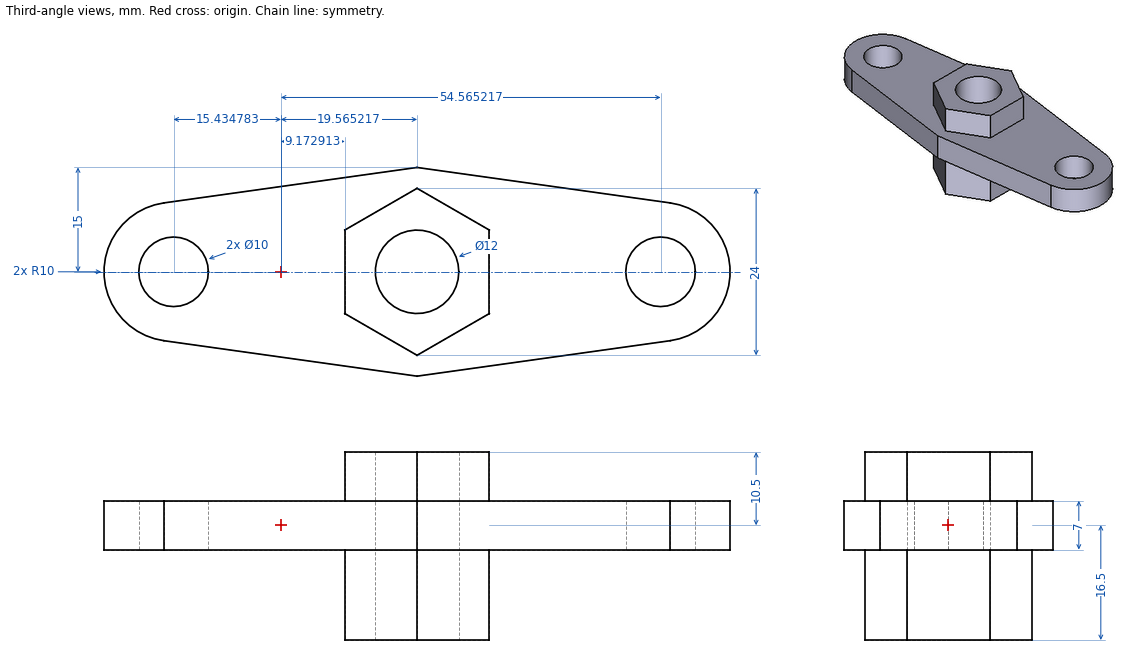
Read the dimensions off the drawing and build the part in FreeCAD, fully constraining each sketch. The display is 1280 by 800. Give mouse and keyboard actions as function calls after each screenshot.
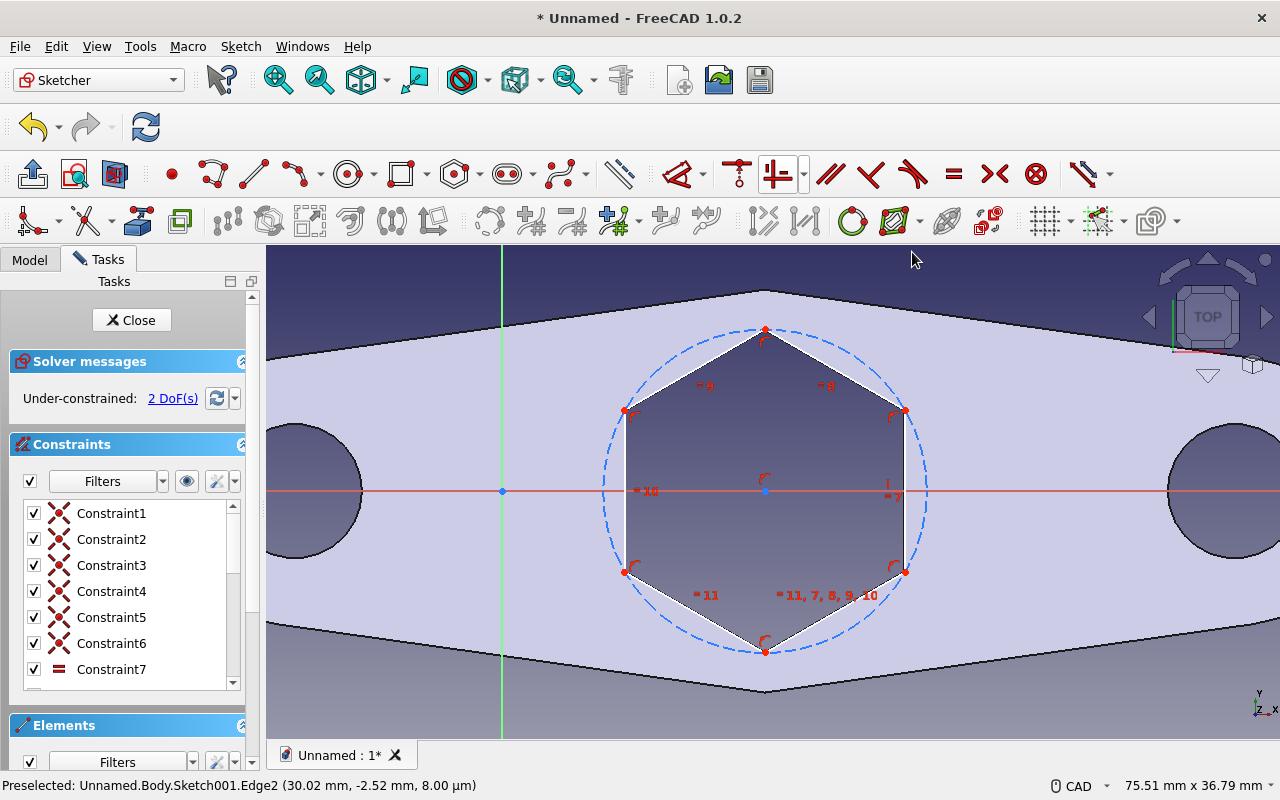
click(676, 174)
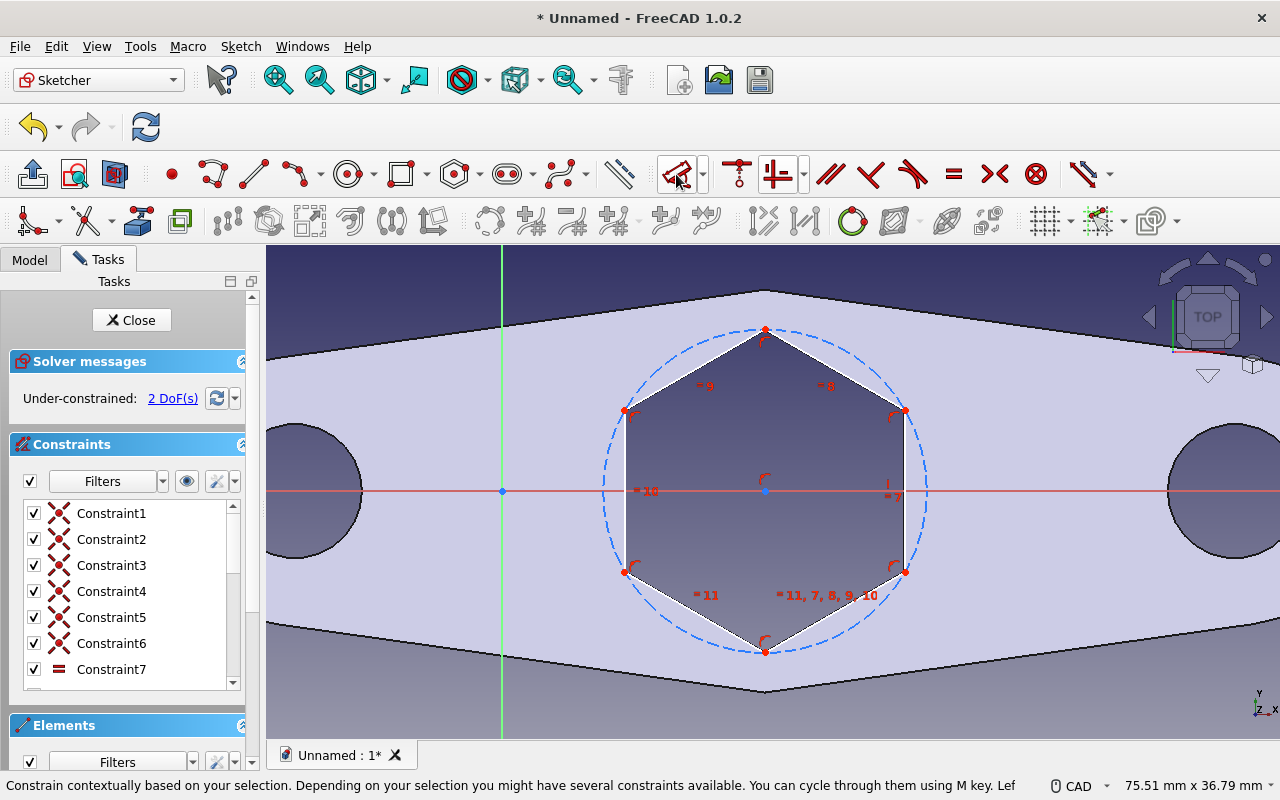
click(765, 653)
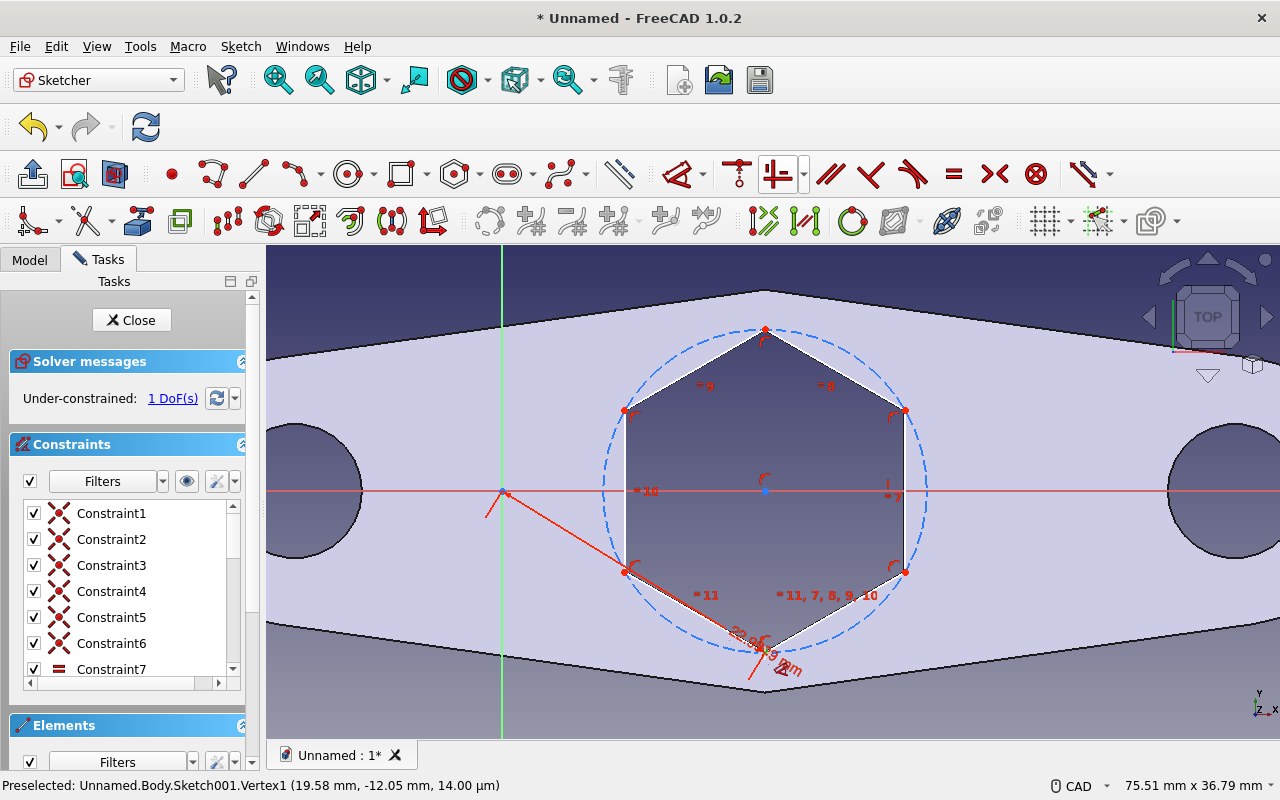
click(765, 329)
click(799, 417)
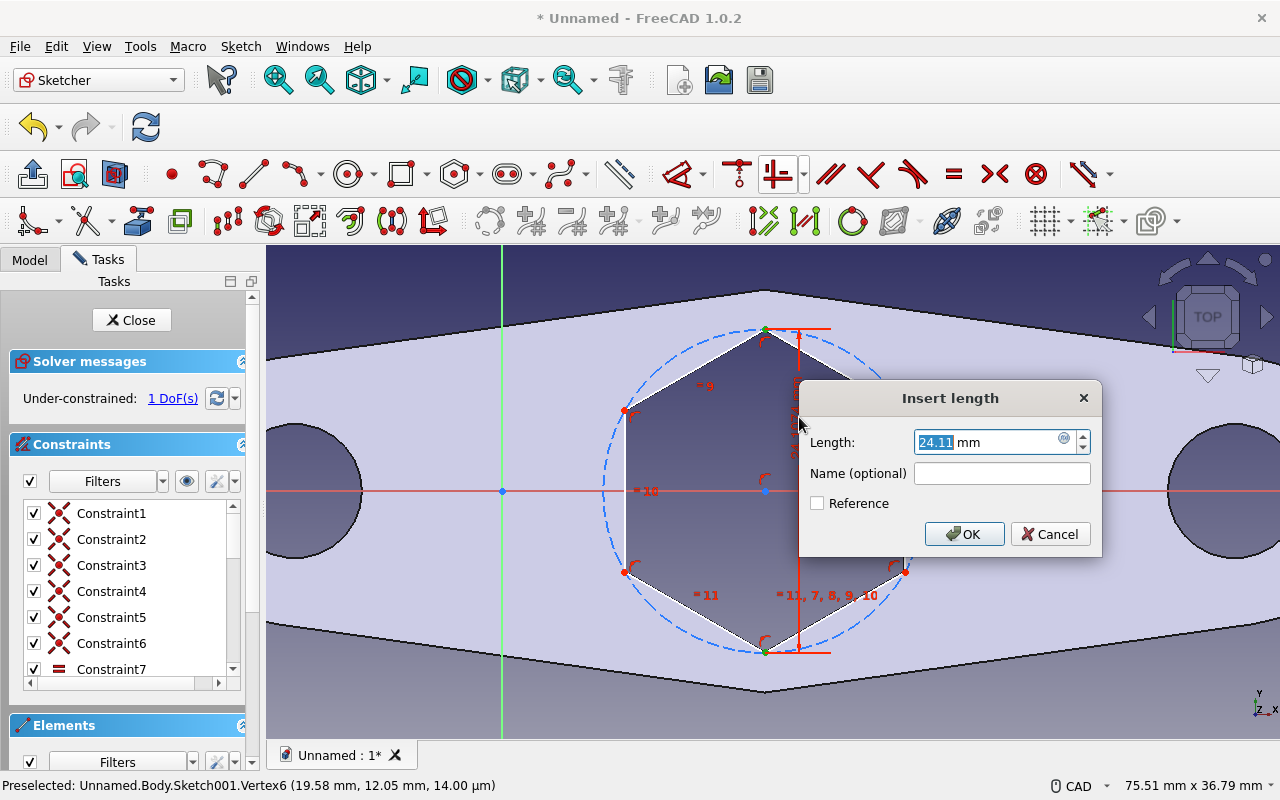
text(24)
key(Return)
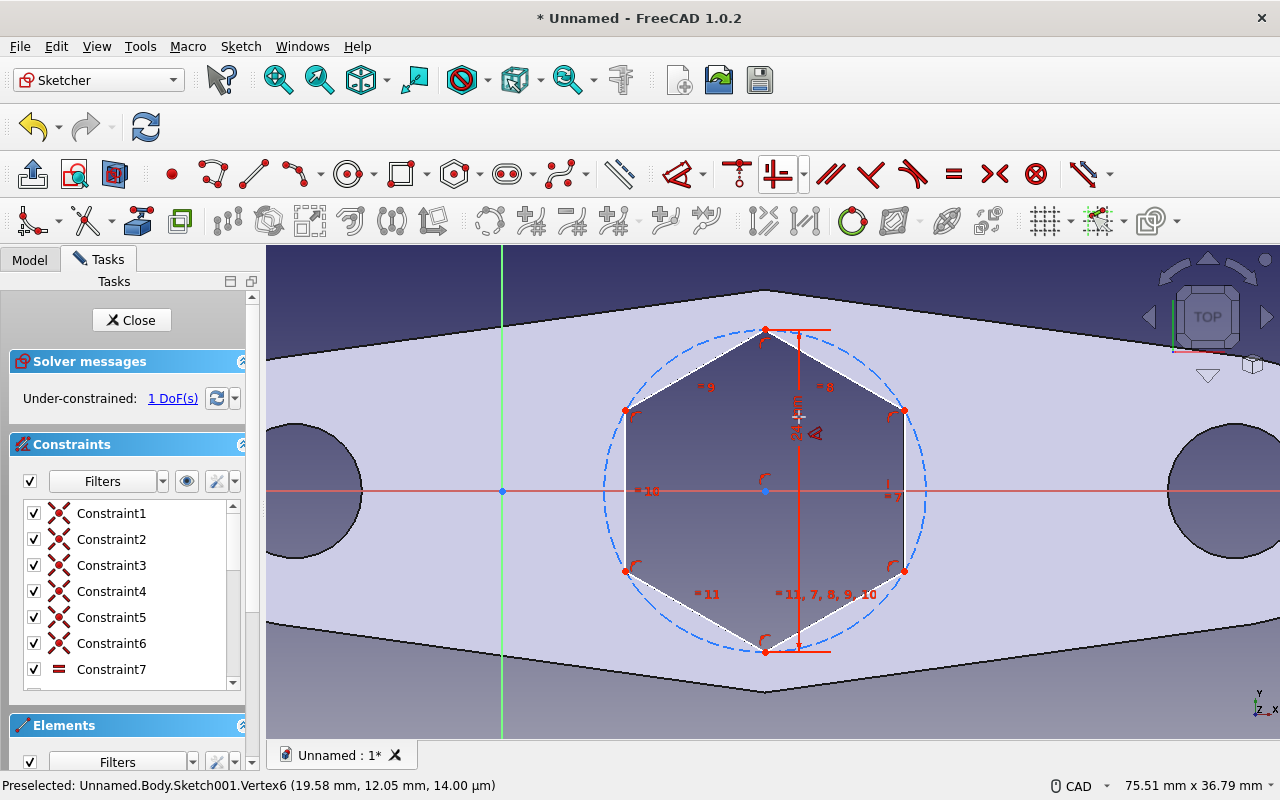
click(625, 411)
click(564, 377)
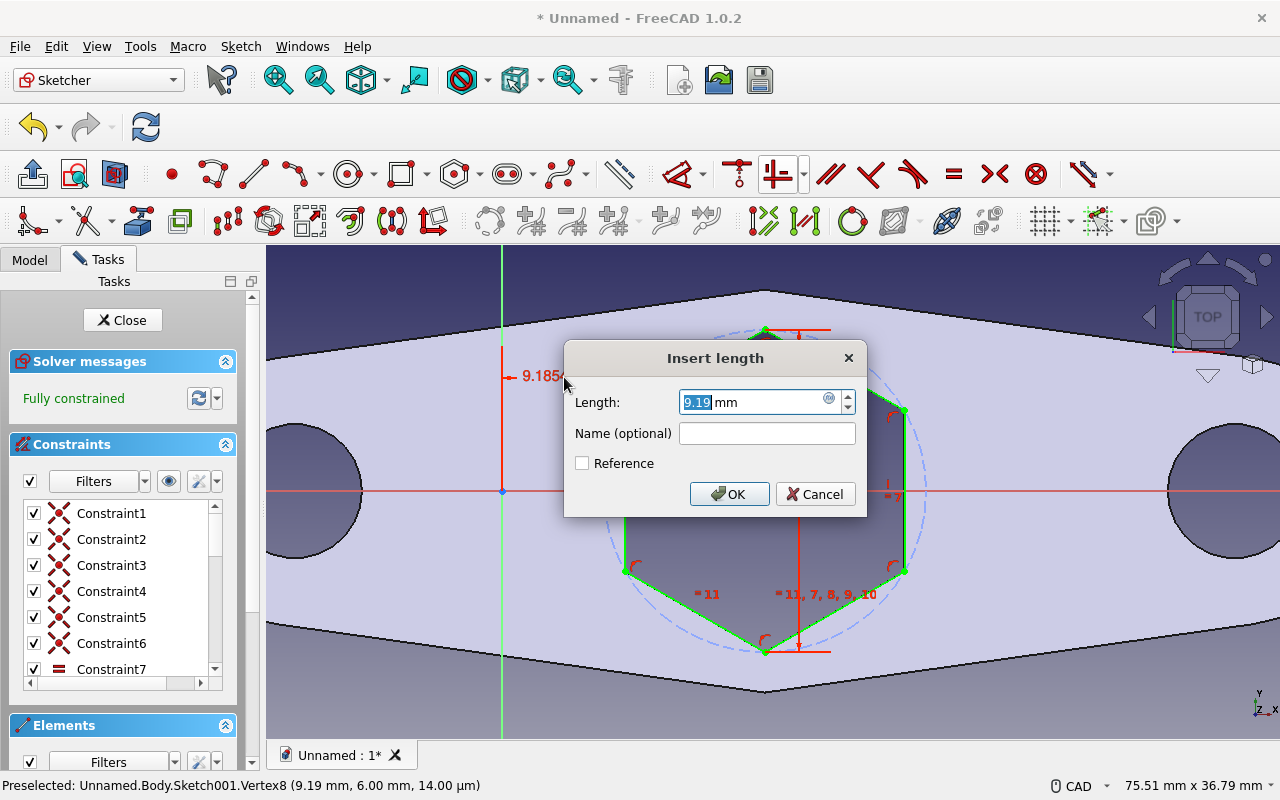
text(9.172913)
key(Return)
key(Escape)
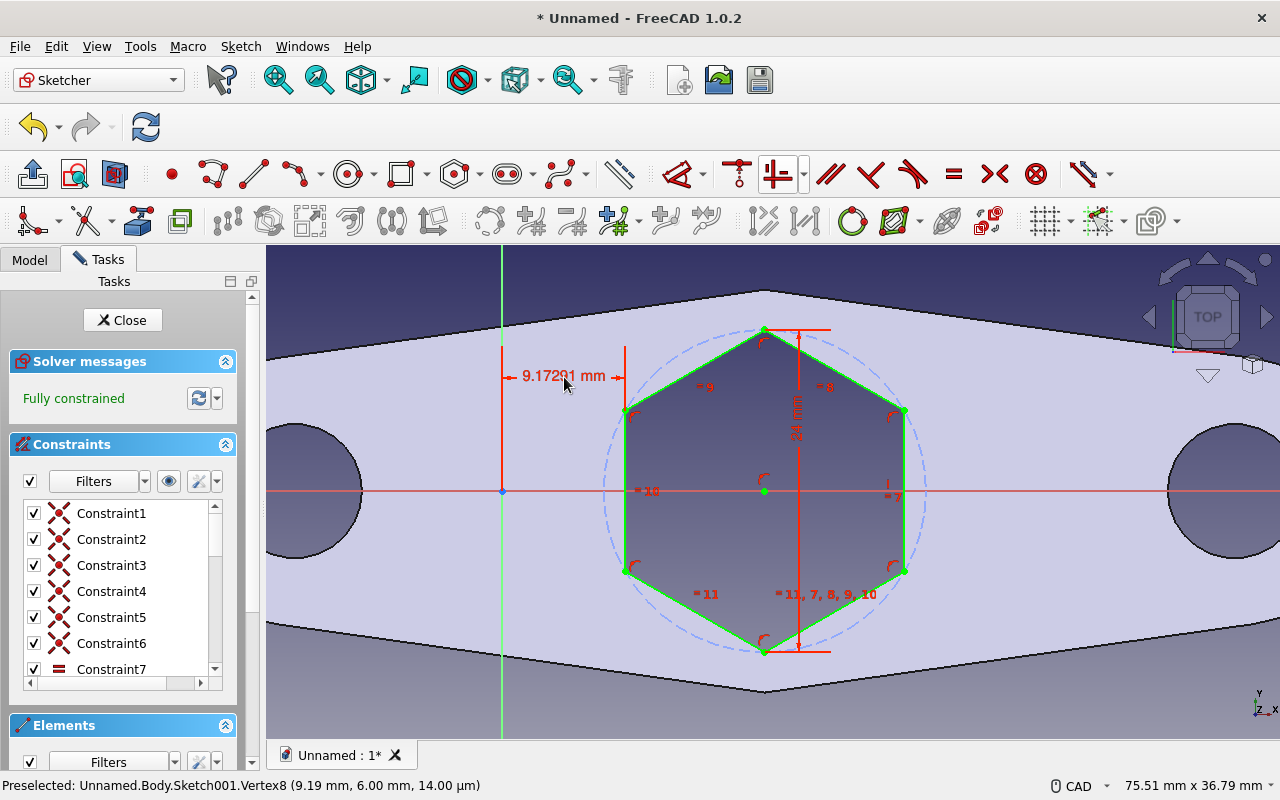
click(123, 320)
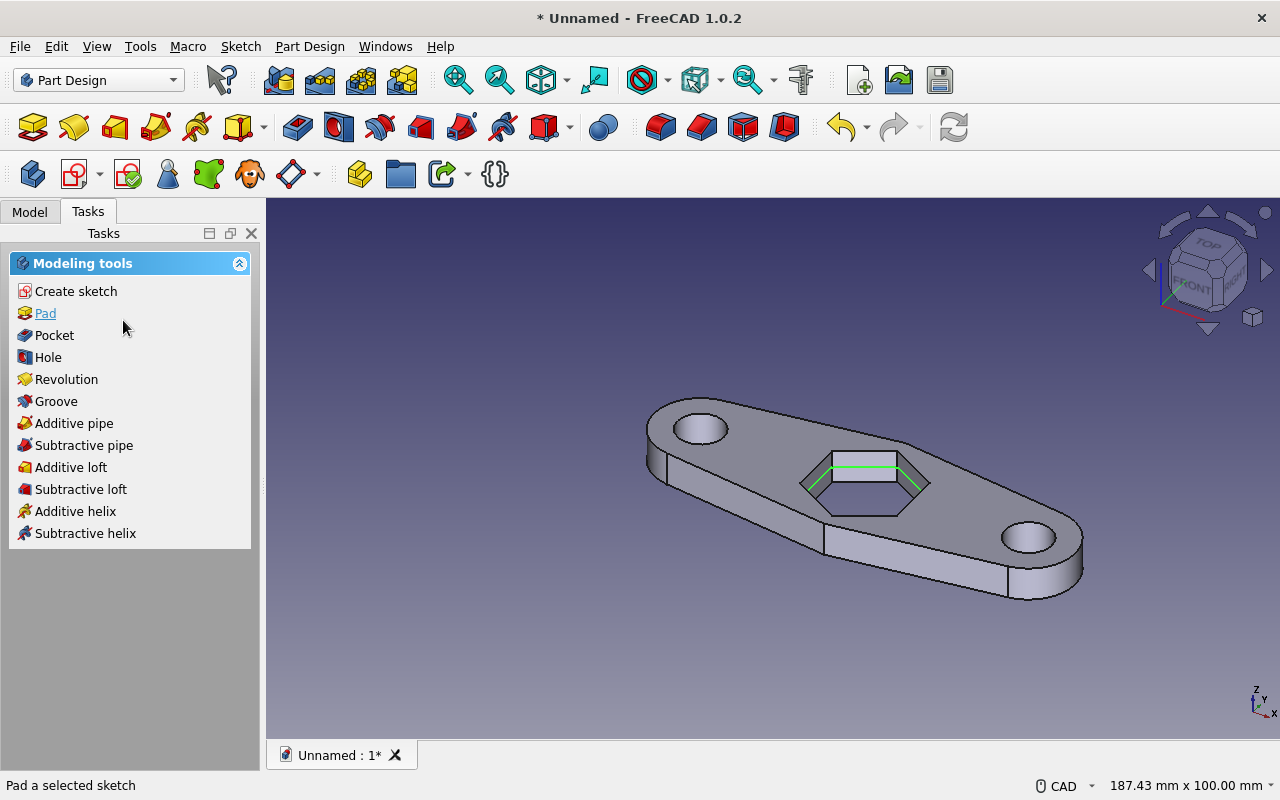
click(33, 128)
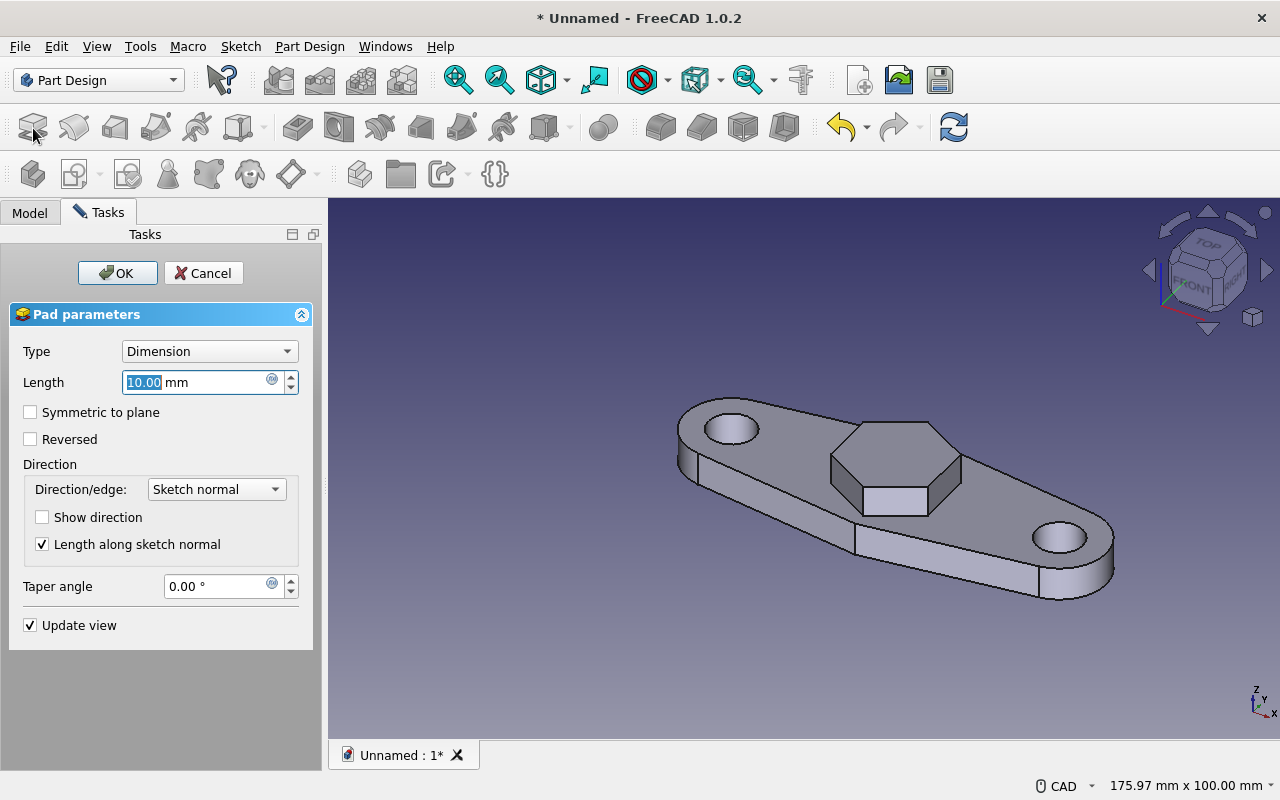
text(10.5)
key(Tab)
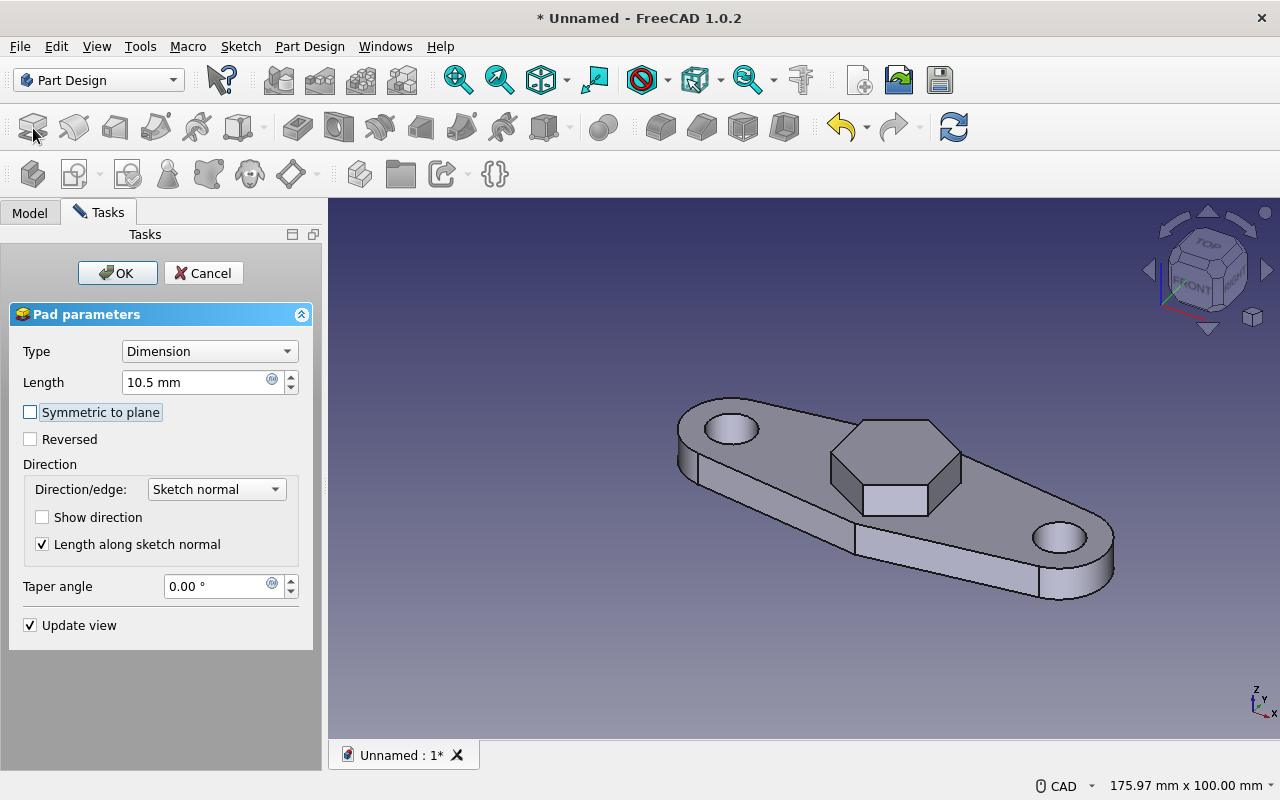
click(118, 273)